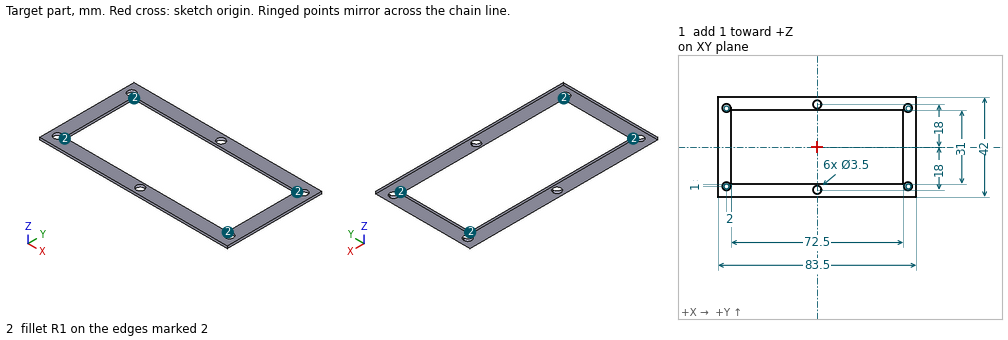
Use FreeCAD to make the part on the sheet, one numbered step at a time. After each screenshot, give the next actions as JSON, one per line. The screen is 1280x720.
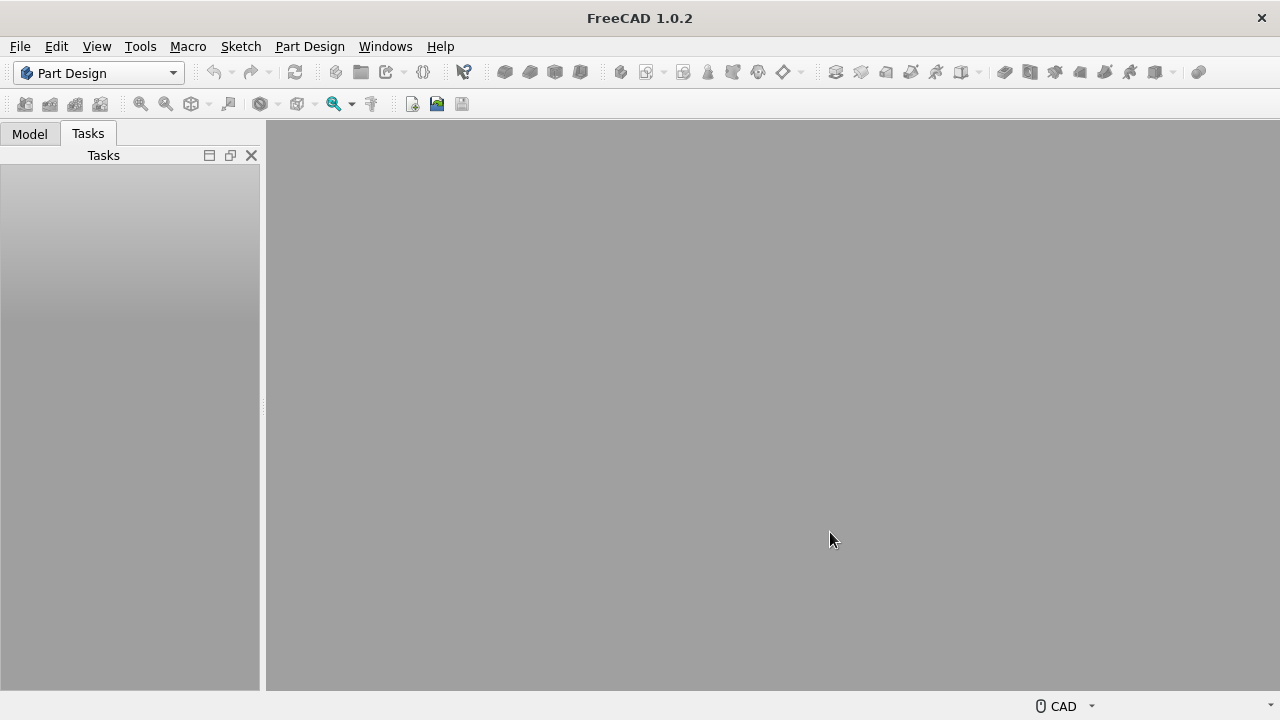
{"action": "left_click", "coordinate": [412, 104]}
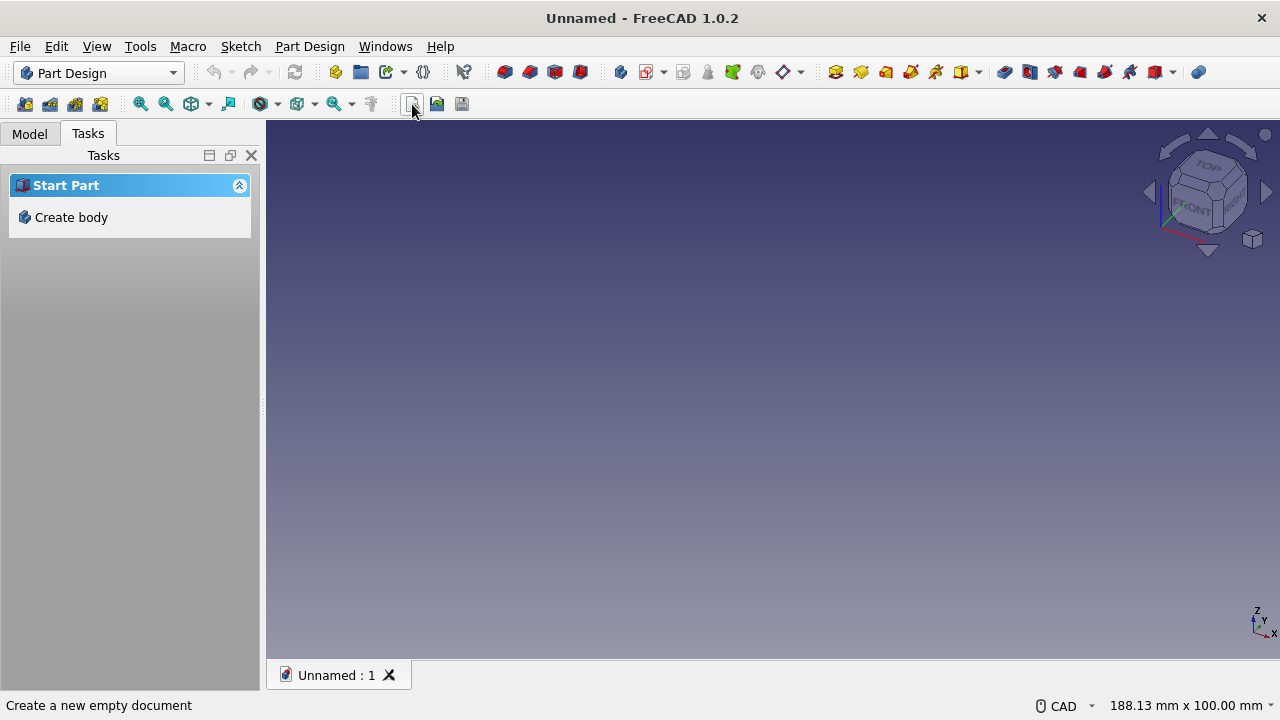
{"action": "left_click", "coordinate": [646, 72]}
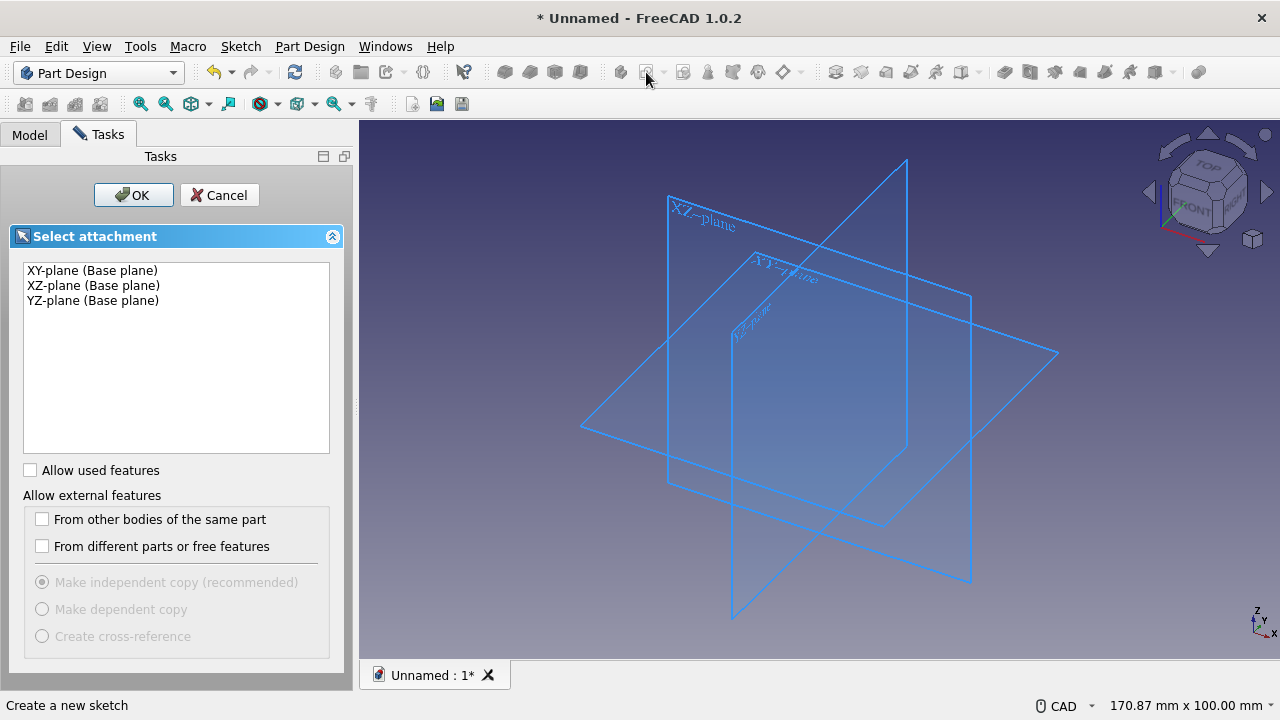
{"action": "left_click", "coordinate": [84, 270]}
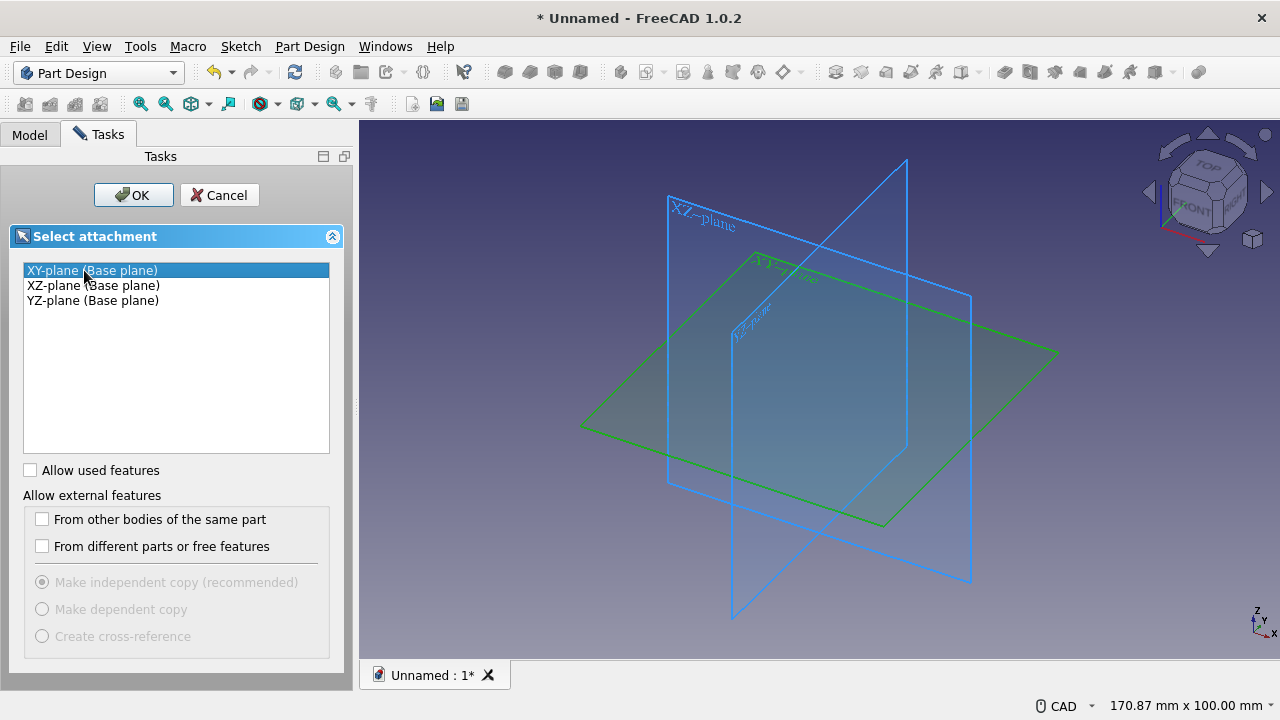
{"action": "left_click", "coordinate": [134, 195]}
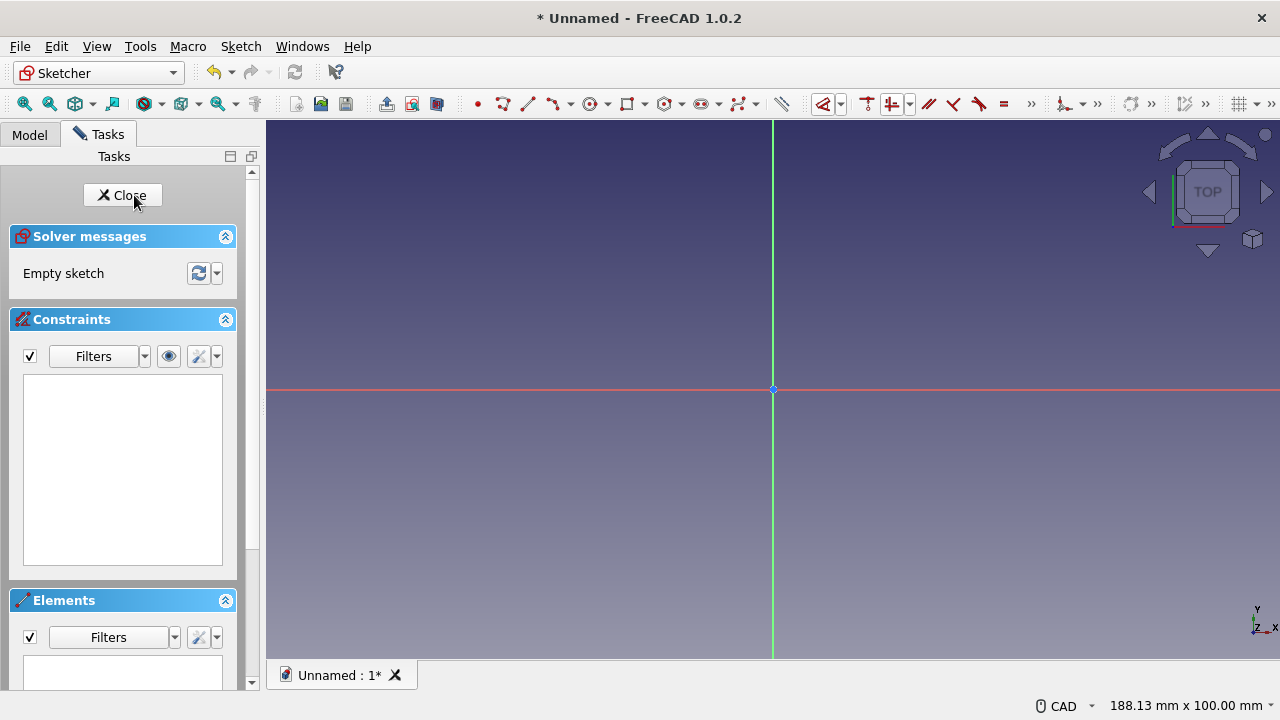
{"action": "key", "text": "g v"}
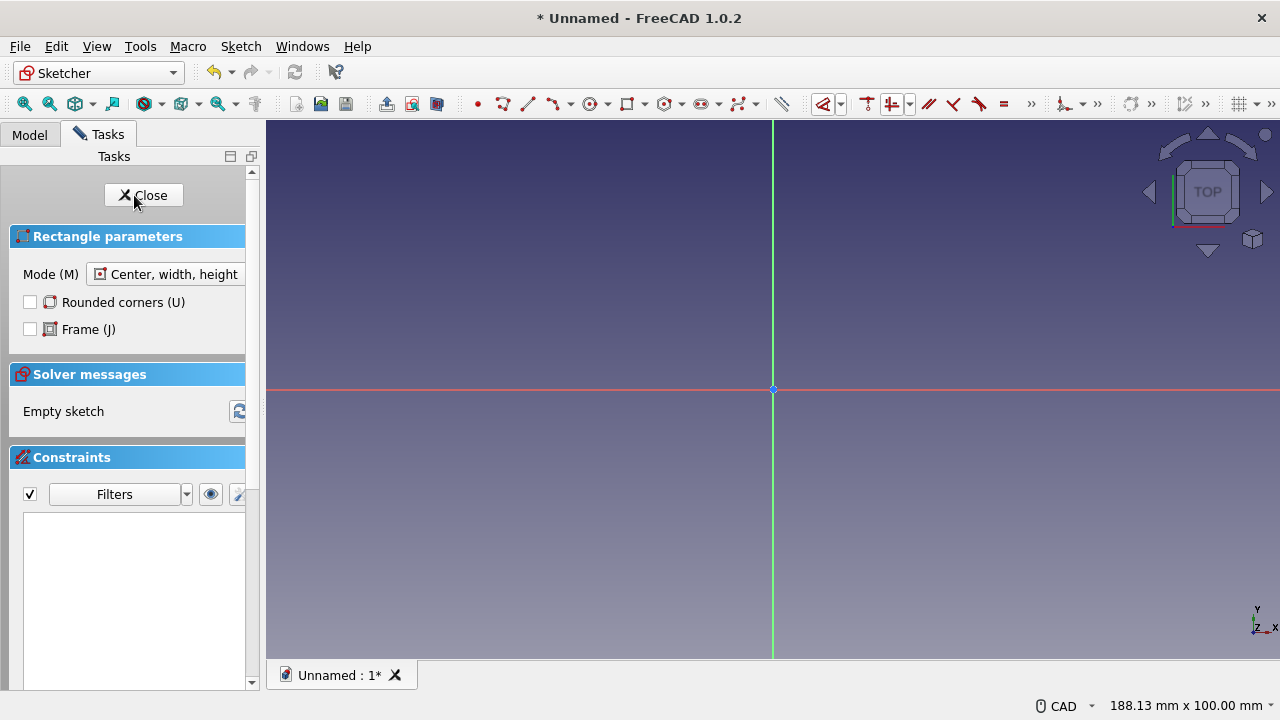
{"action": "left_click", "coordinate": [773, 390]}
{"action": "mouse_move", "coordinate": [998, 276]}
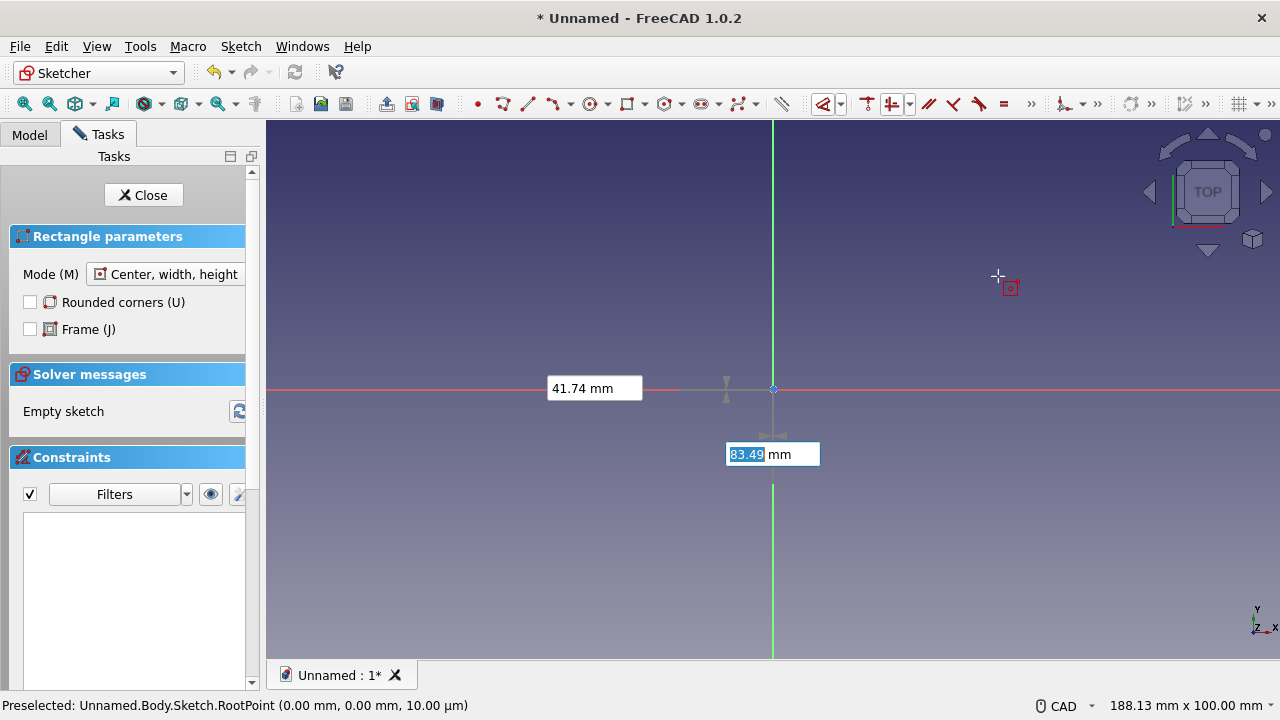
{"action": "type", "text": "83.5"}
{"action": "key", "text": "Tab"}
{"action": "type", "text": "42"}
{"action": "key", "text": "Return"}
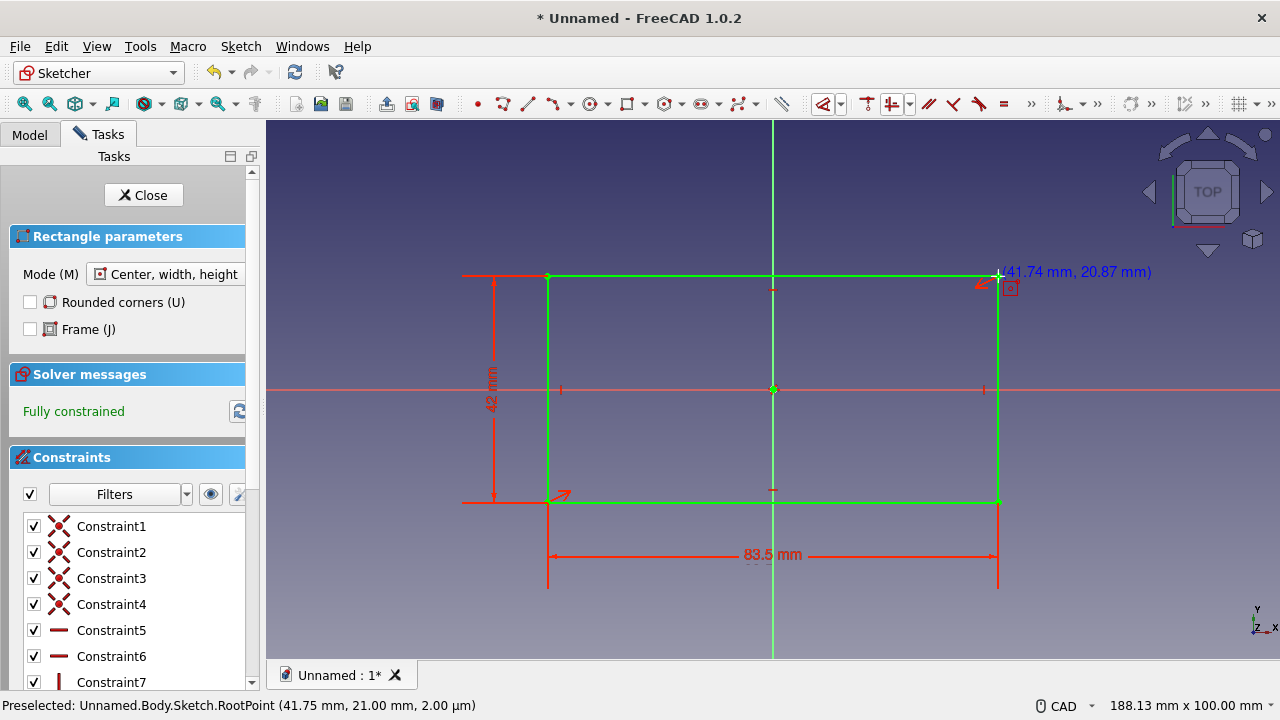
{"action": "left_click", "coordinate": [773, 390]}
{"action": "mouse_move", "coordinate": [968, 306]}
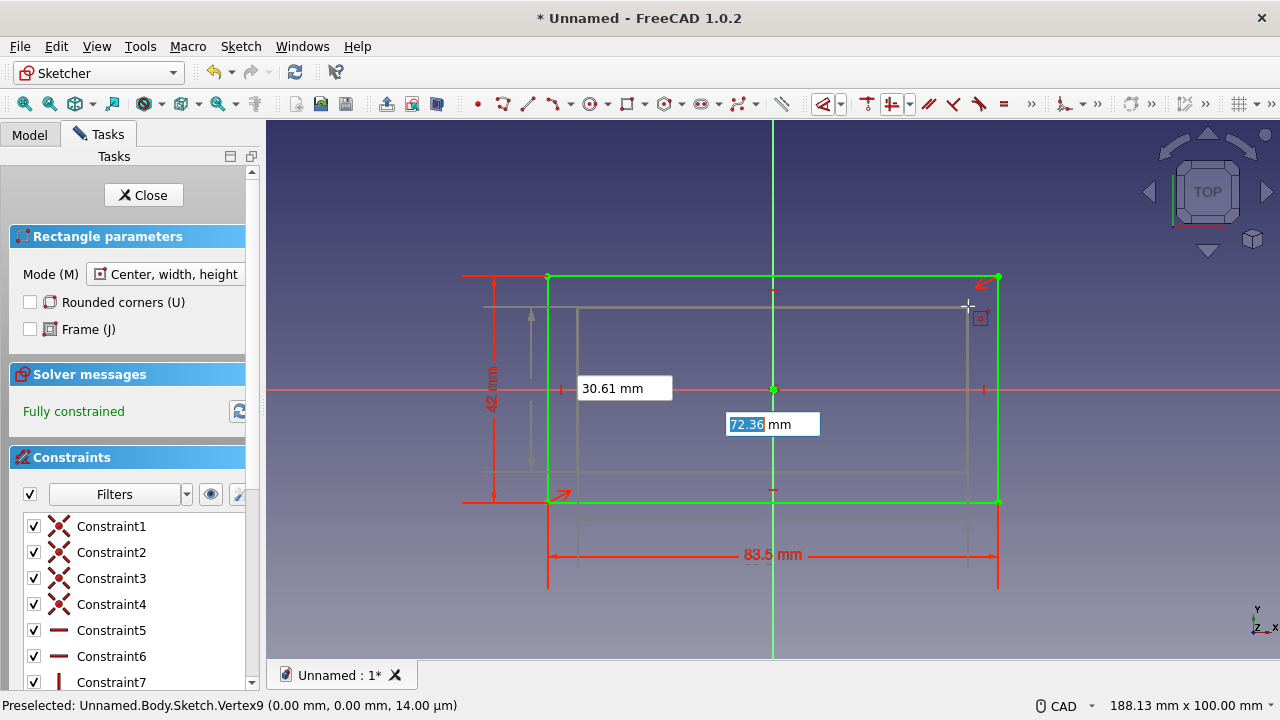
{"action": "type", "text": "72.5"}
{"action": "key", "text": "Tab"}
{"action": "type", "text": "31"}
{"action": "key", "text": "Return"}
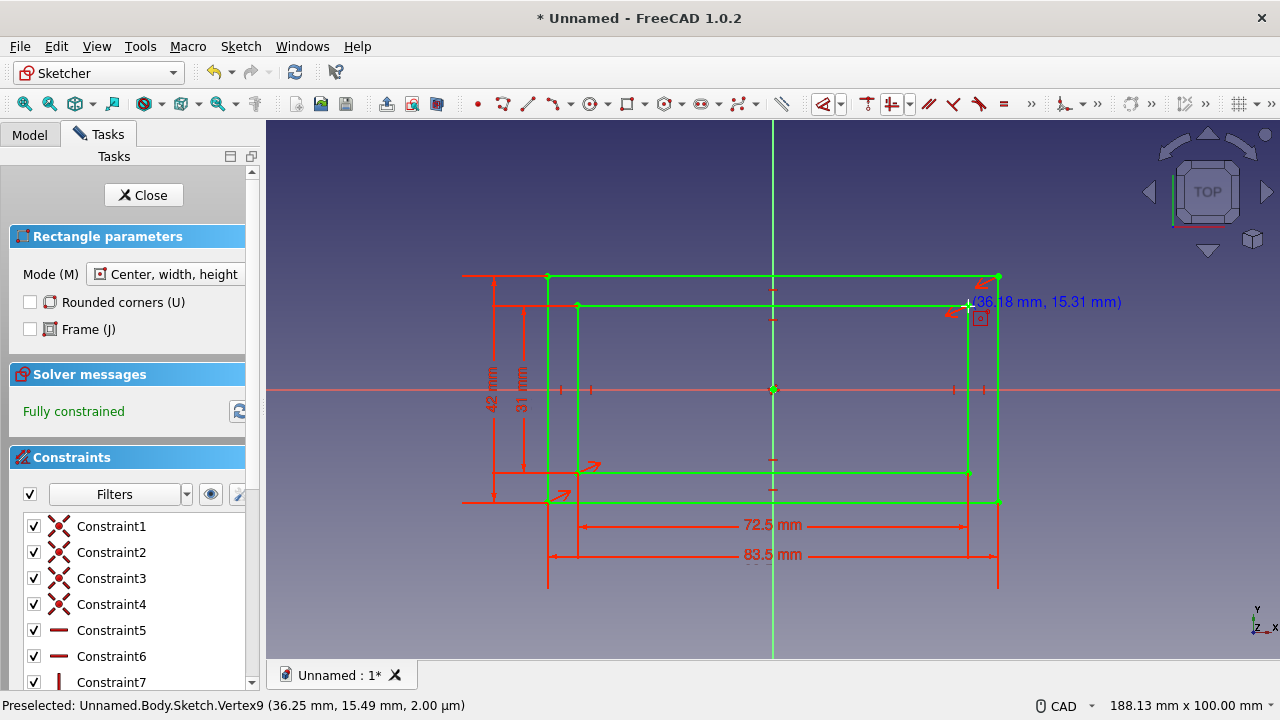
{"action": "left_click", "coordinate": [590, 104]}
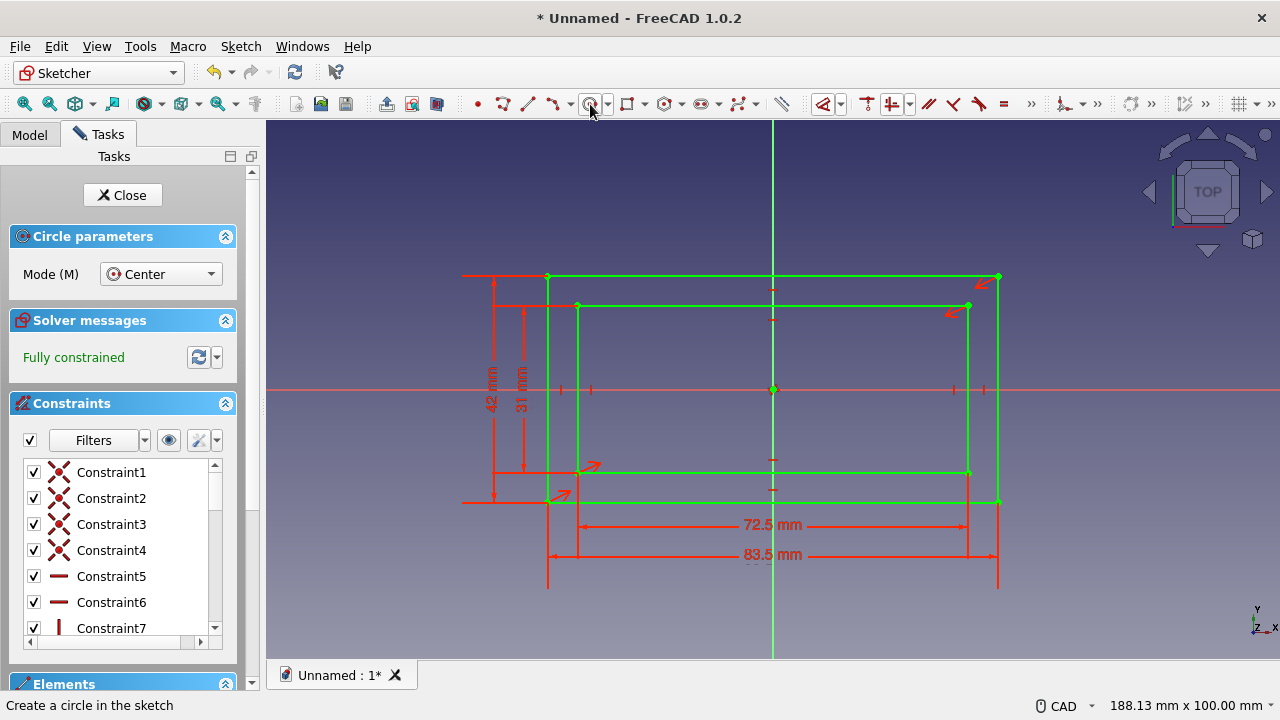
{"action": "scroll", "coordinate": [567, 478], "scroll_direction": "up", "scroll_amount": 5}